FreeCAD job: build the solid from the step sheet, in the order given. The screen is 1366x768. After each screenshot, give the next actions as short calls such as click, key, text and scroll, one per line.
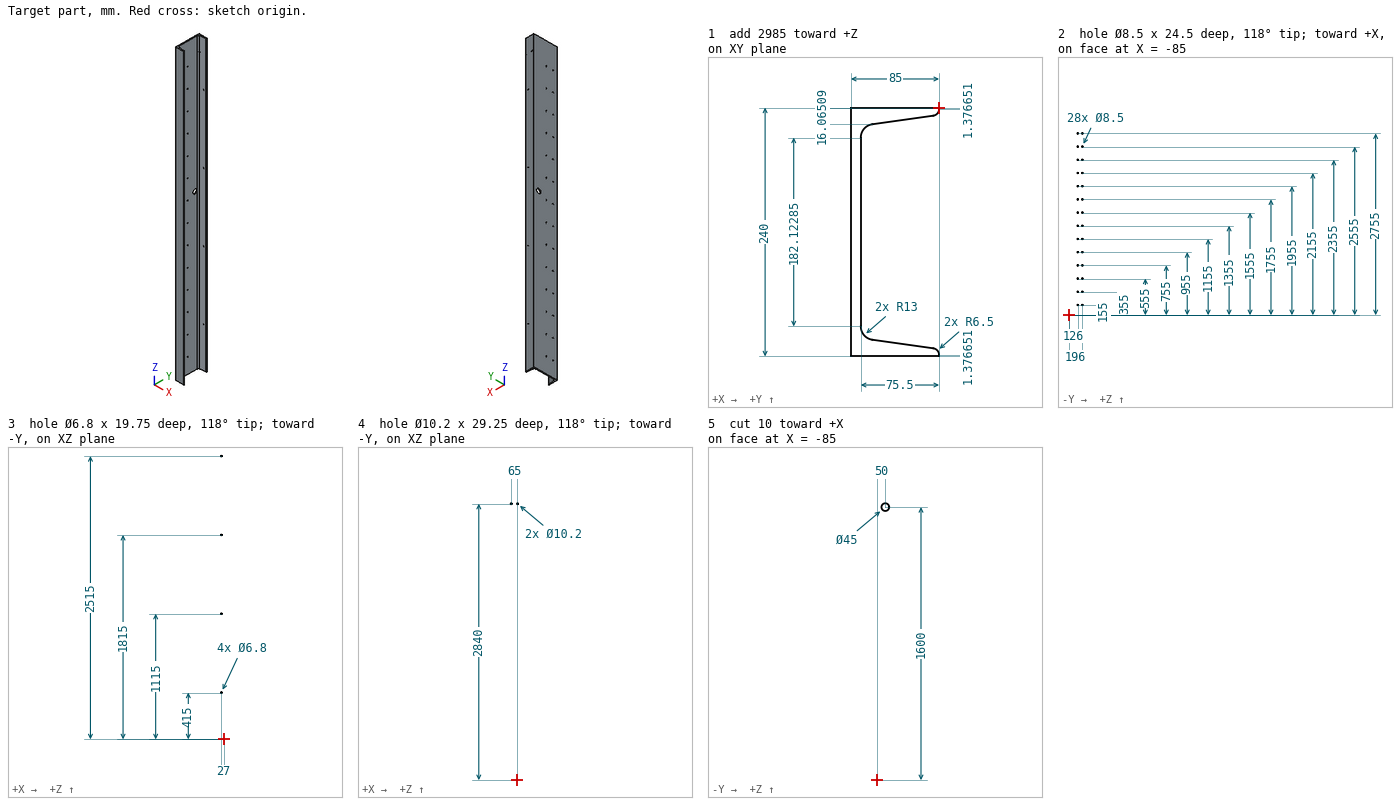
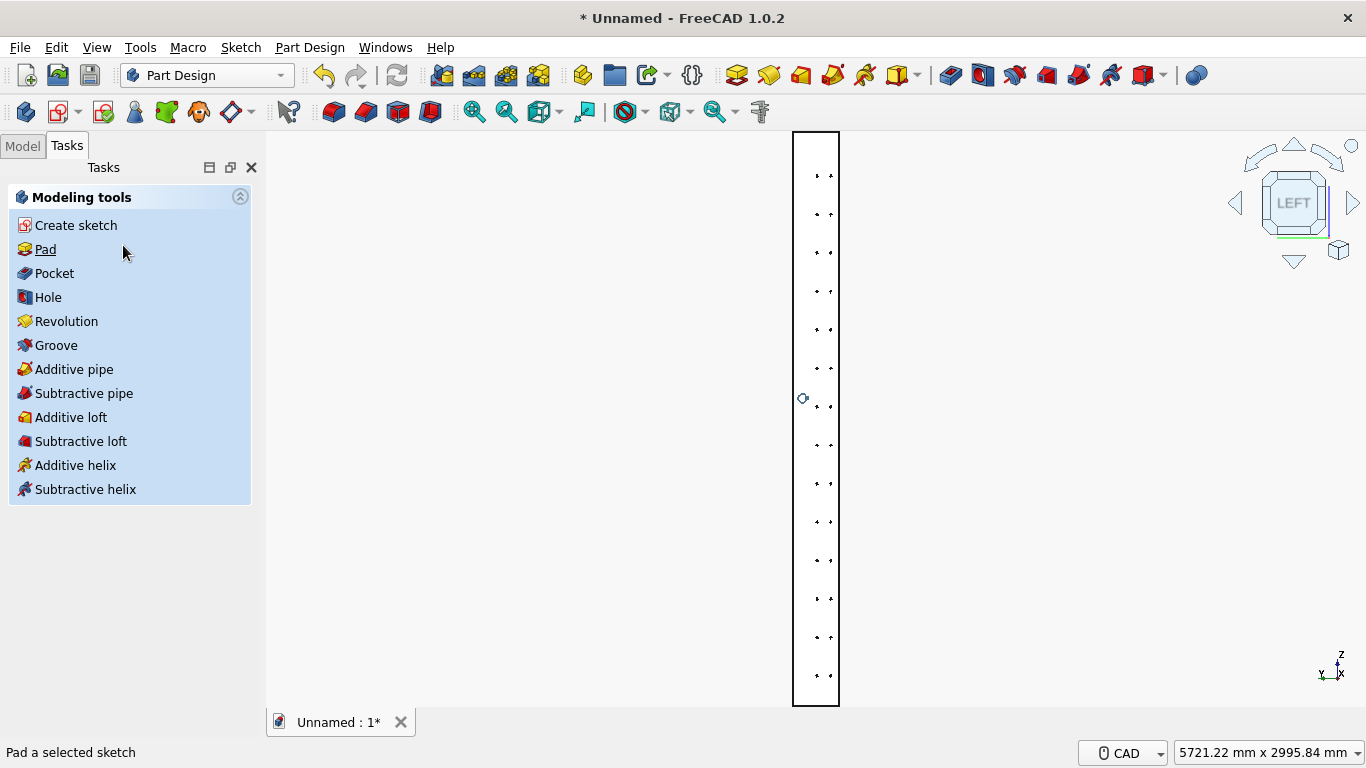
click(952, 76)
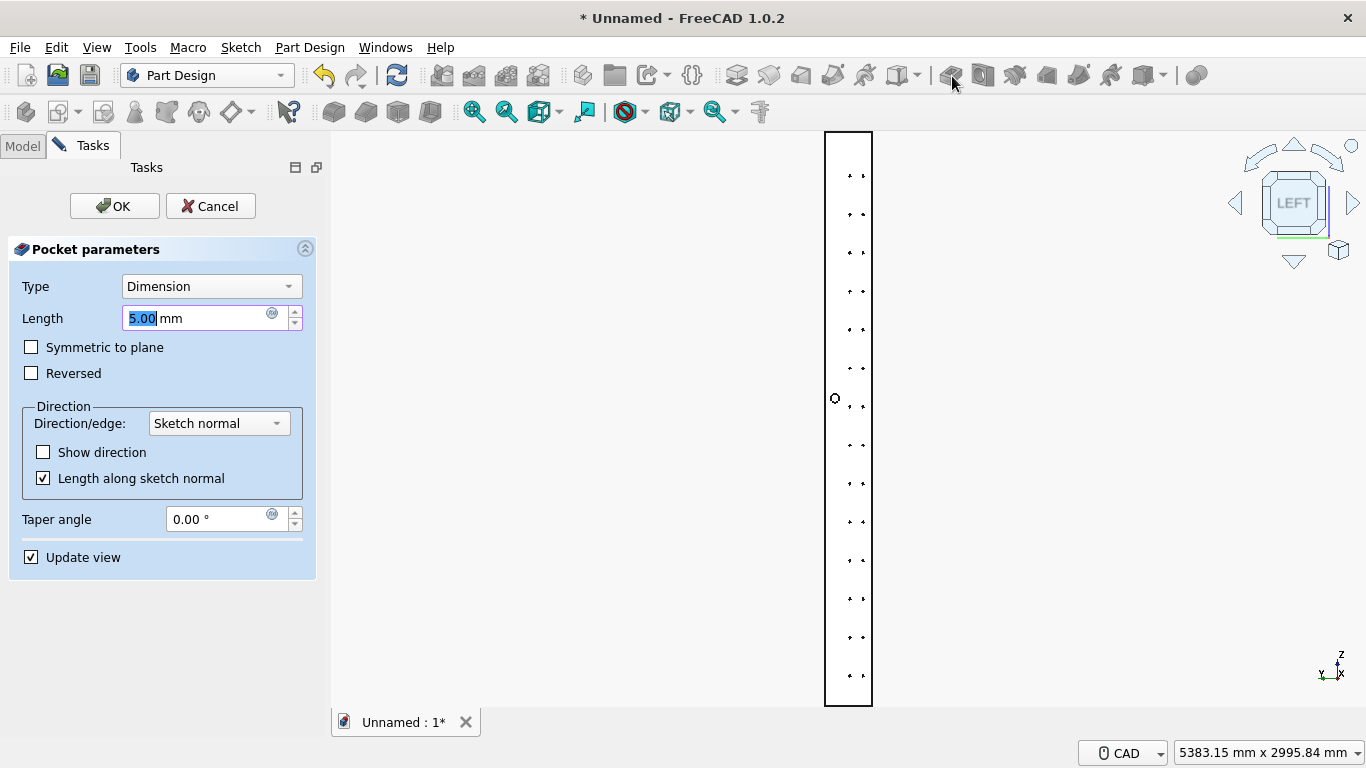
text(10)
key(Tab)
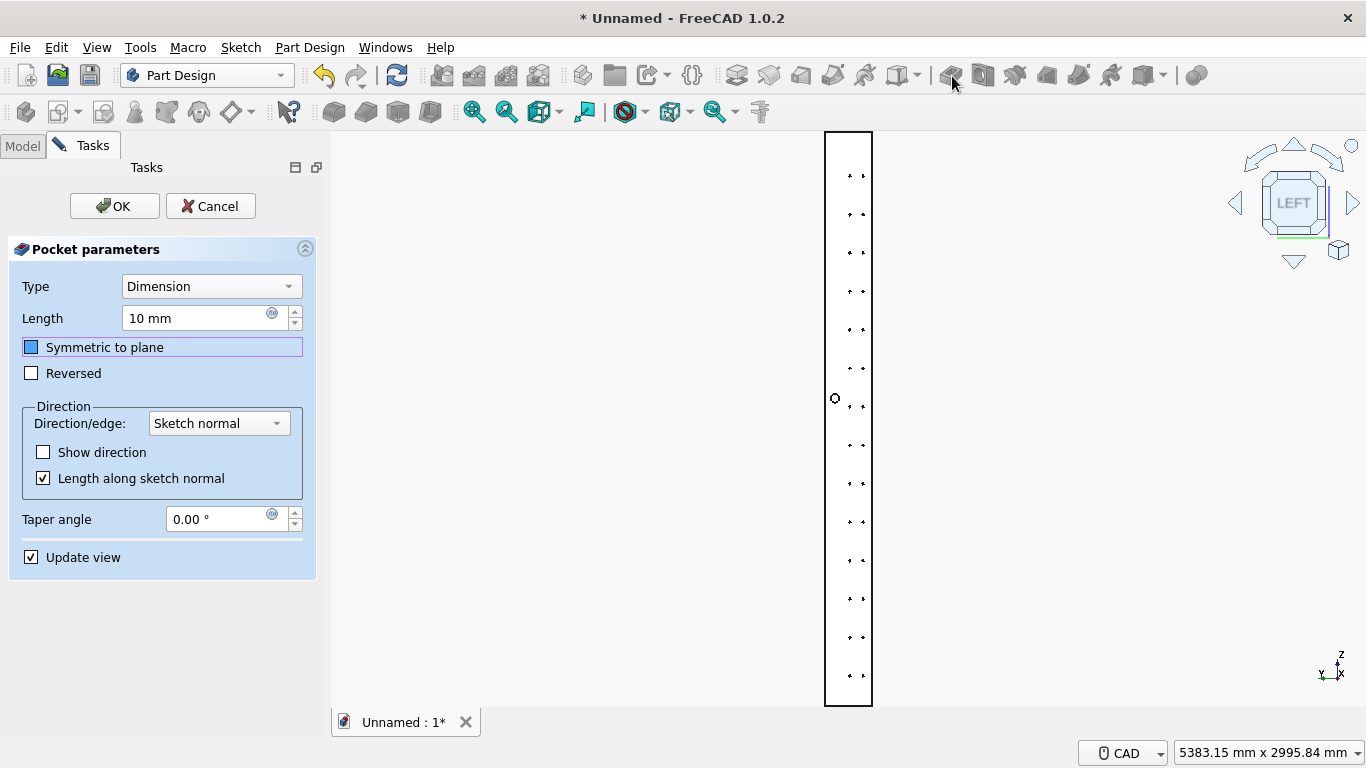
click(115, 206)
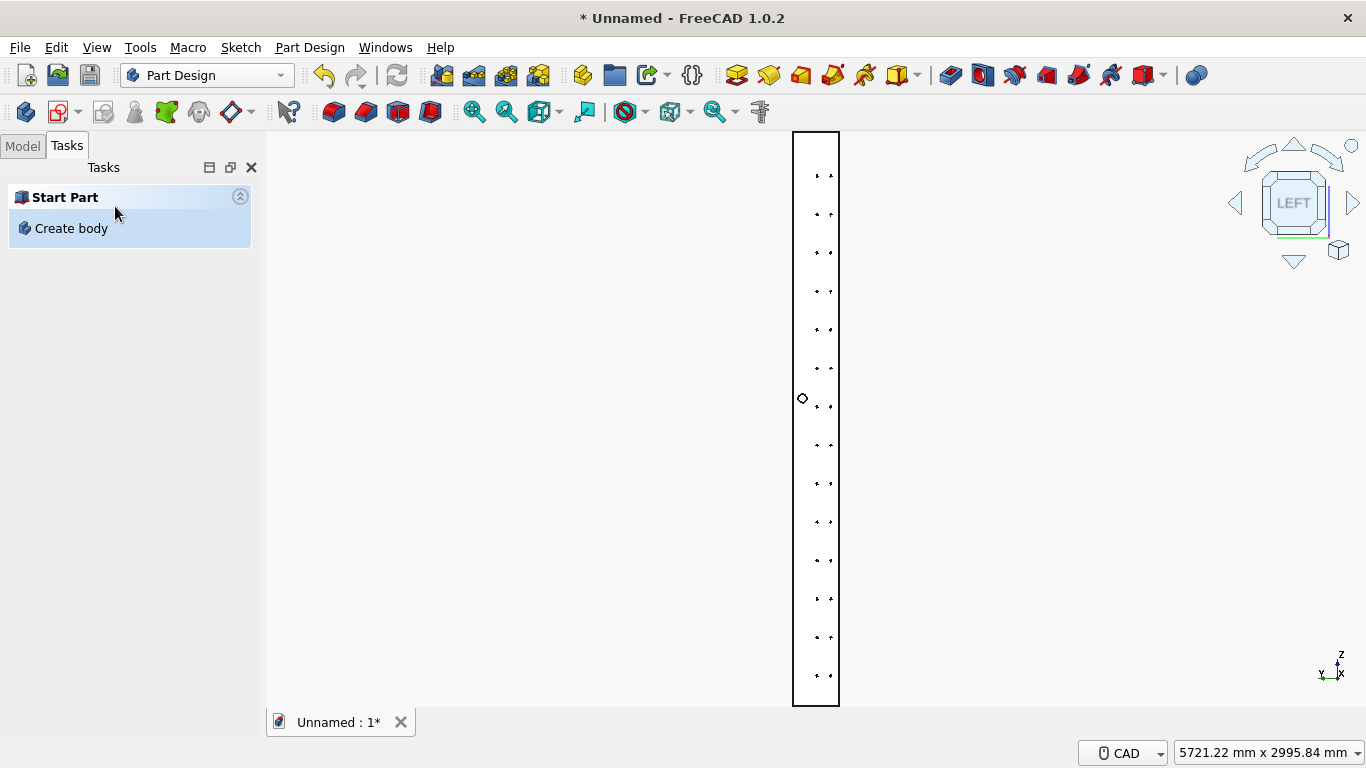
key(0)